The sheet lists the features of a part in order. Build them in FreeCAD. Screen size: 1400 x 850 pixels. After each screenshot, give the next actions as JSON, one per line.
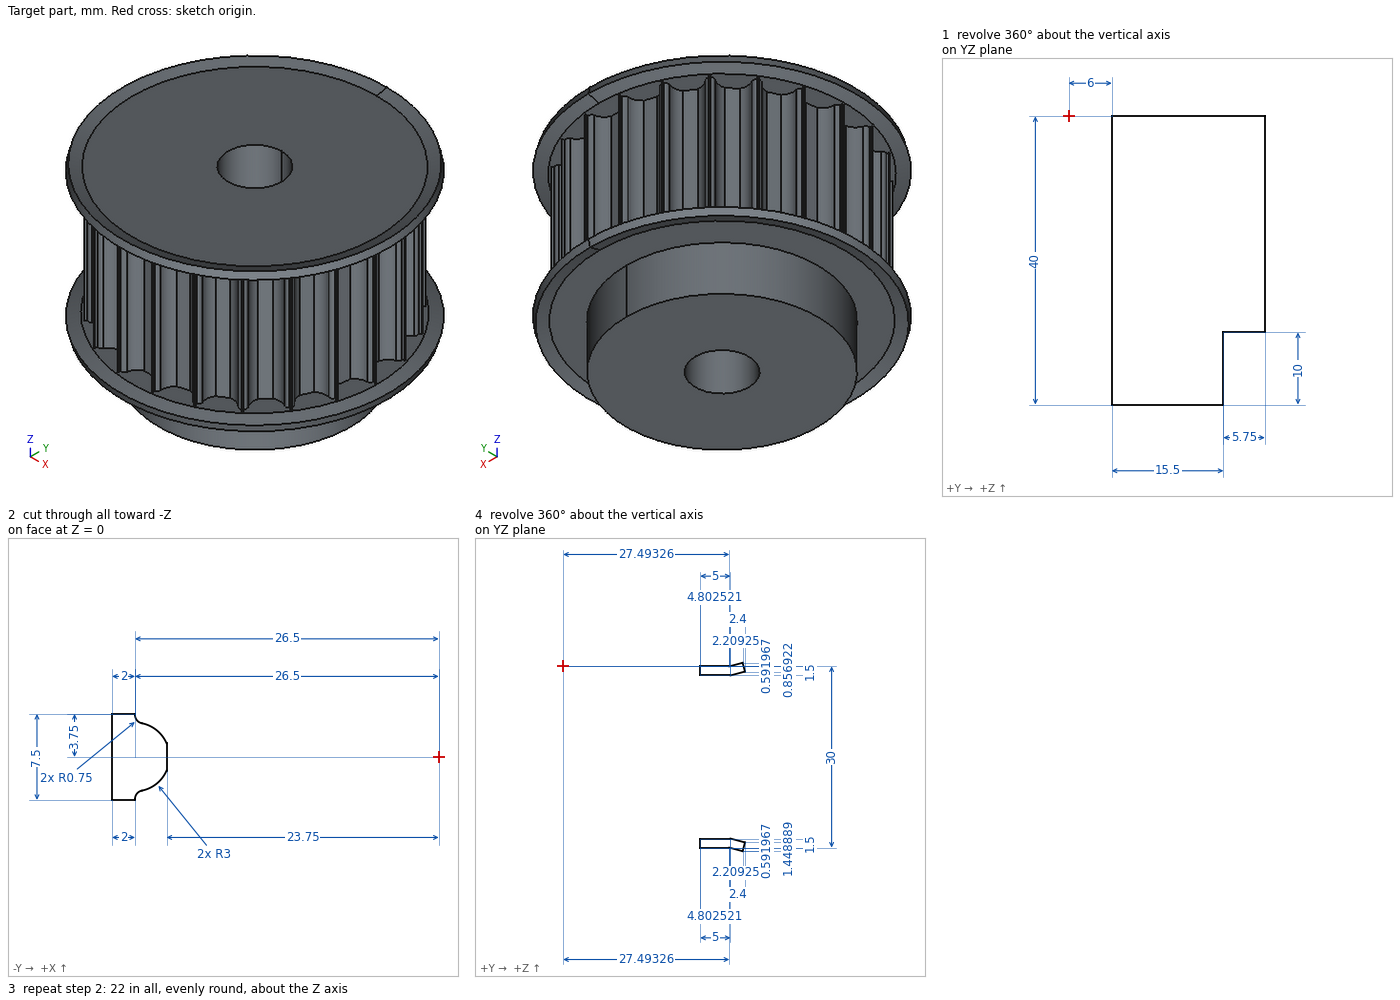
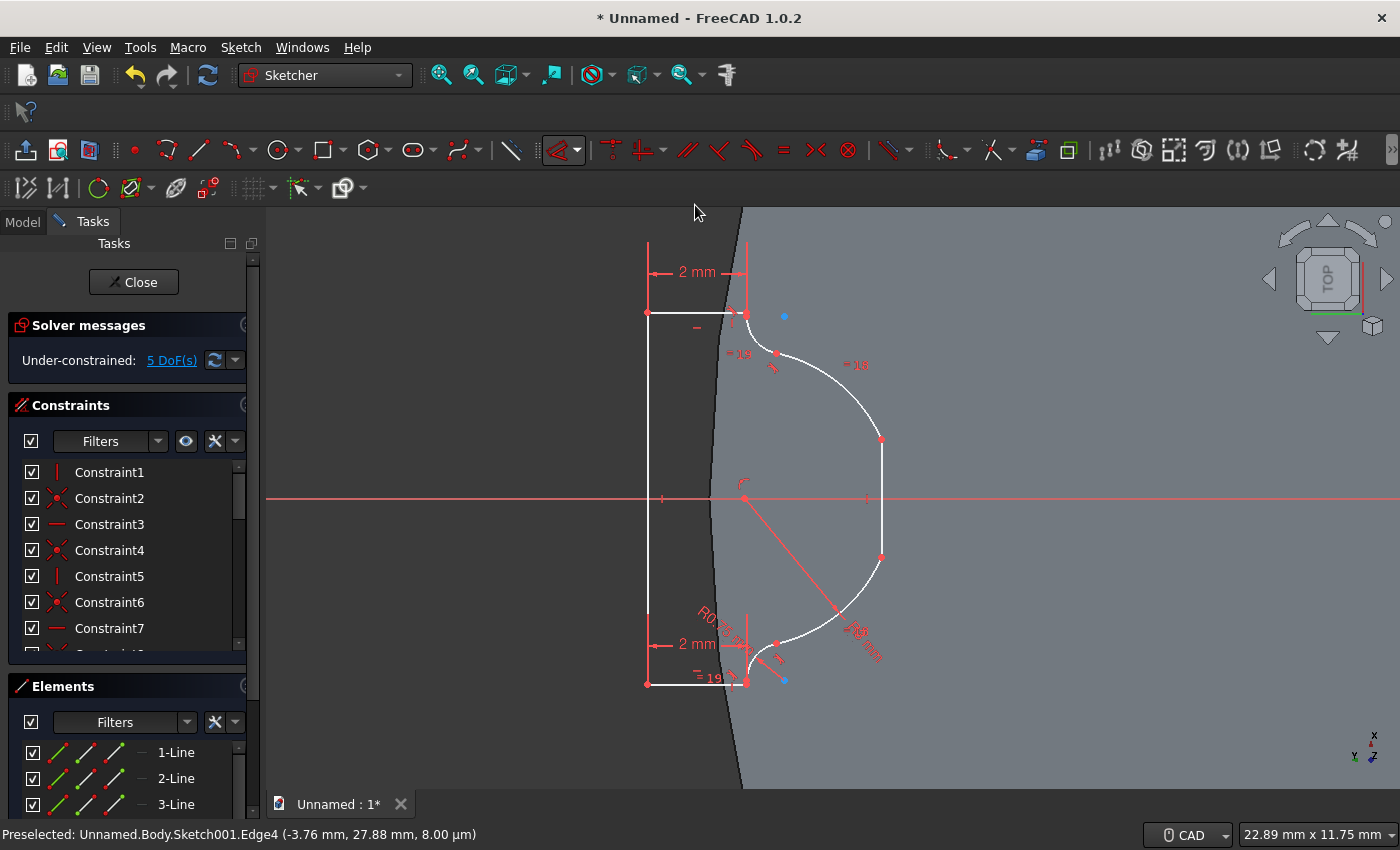
{"action": "left_click", "coordinate": [648, 425]}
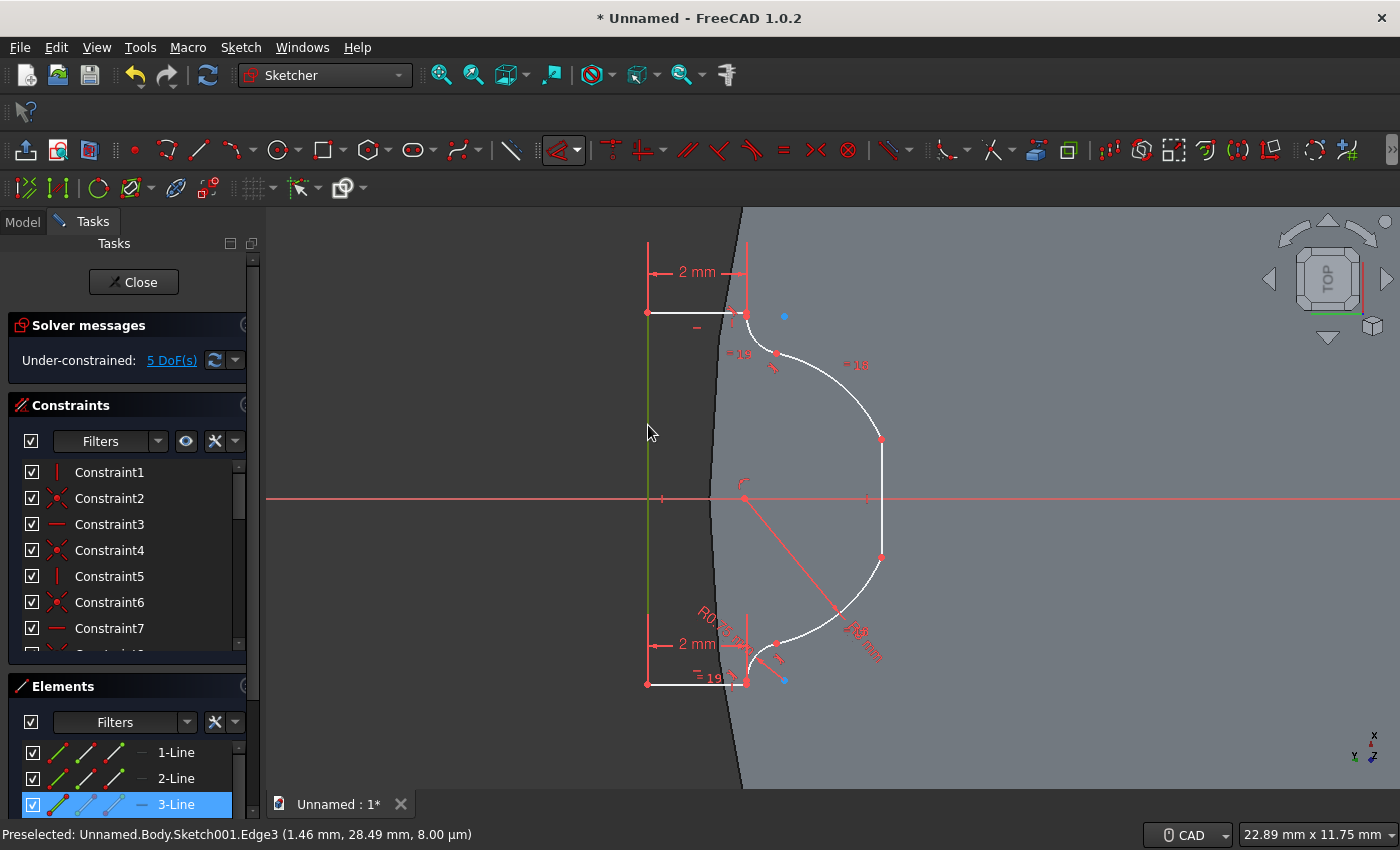
{"action": "key", "text": "i"}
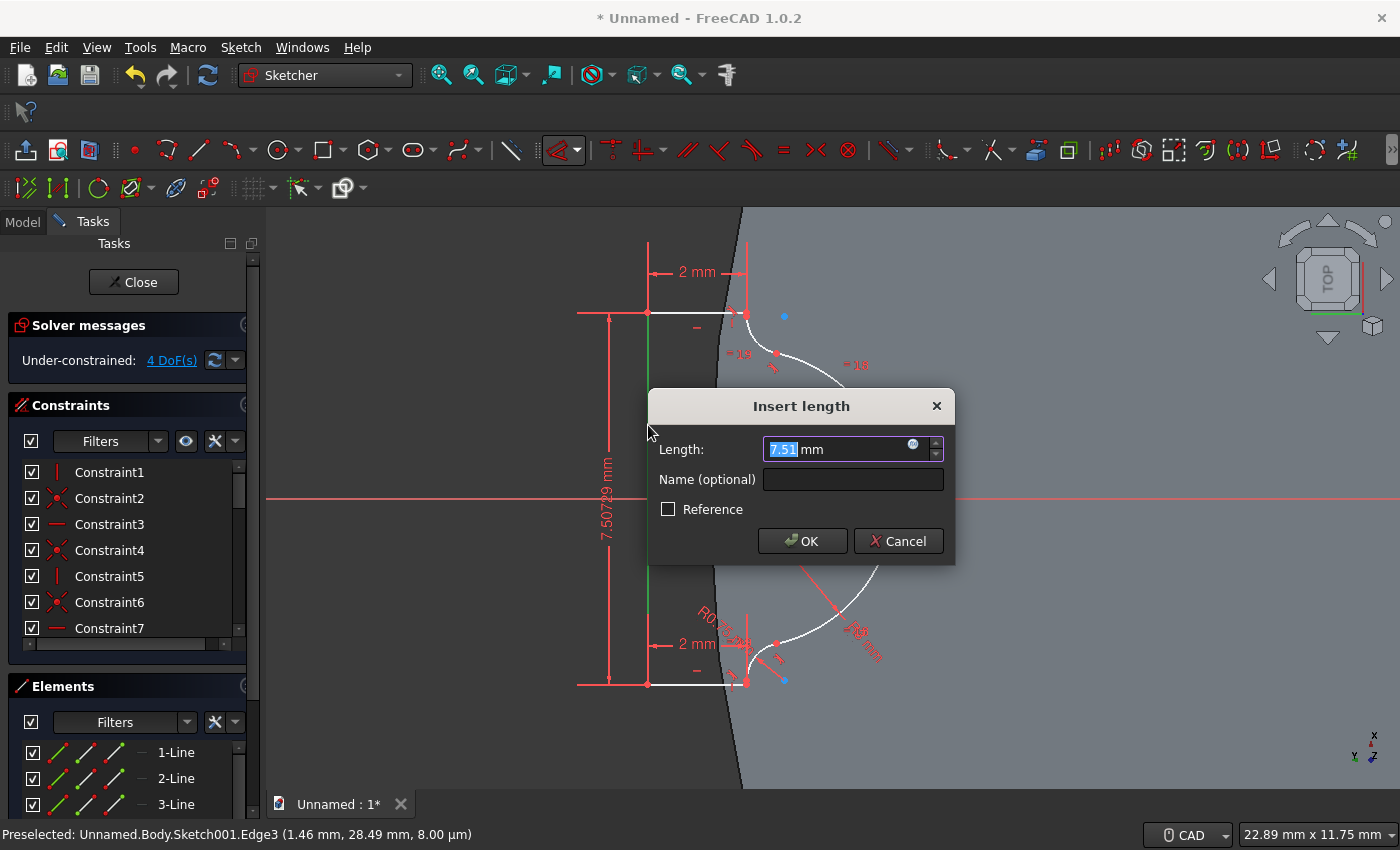
{"action": "type", "text": "7.5"}
{"action": "key", "text": "Return"}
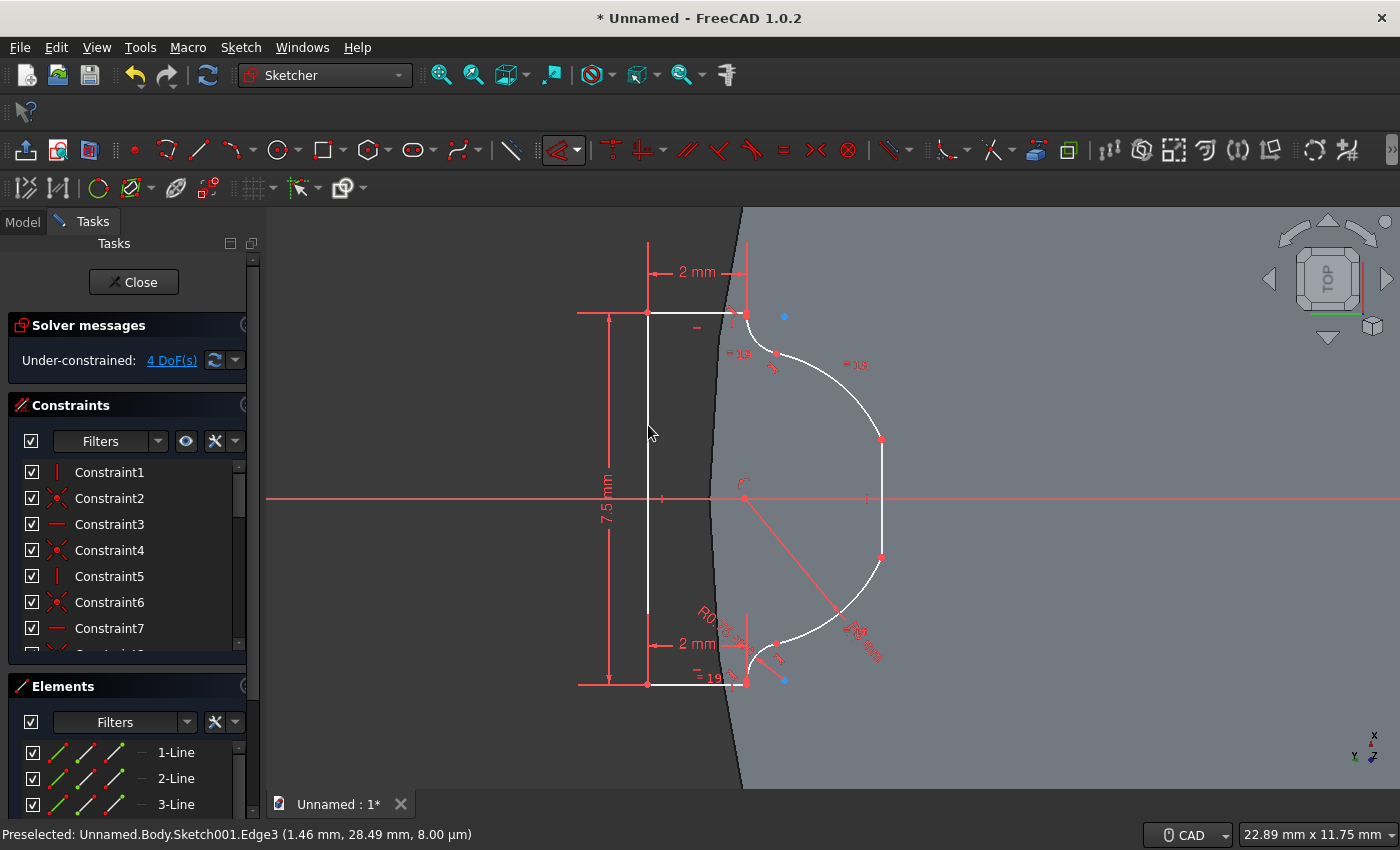
{"action": "scroll", "coordinate": [747, 317], "scroll_direction": "up", "scroll_amount": 6}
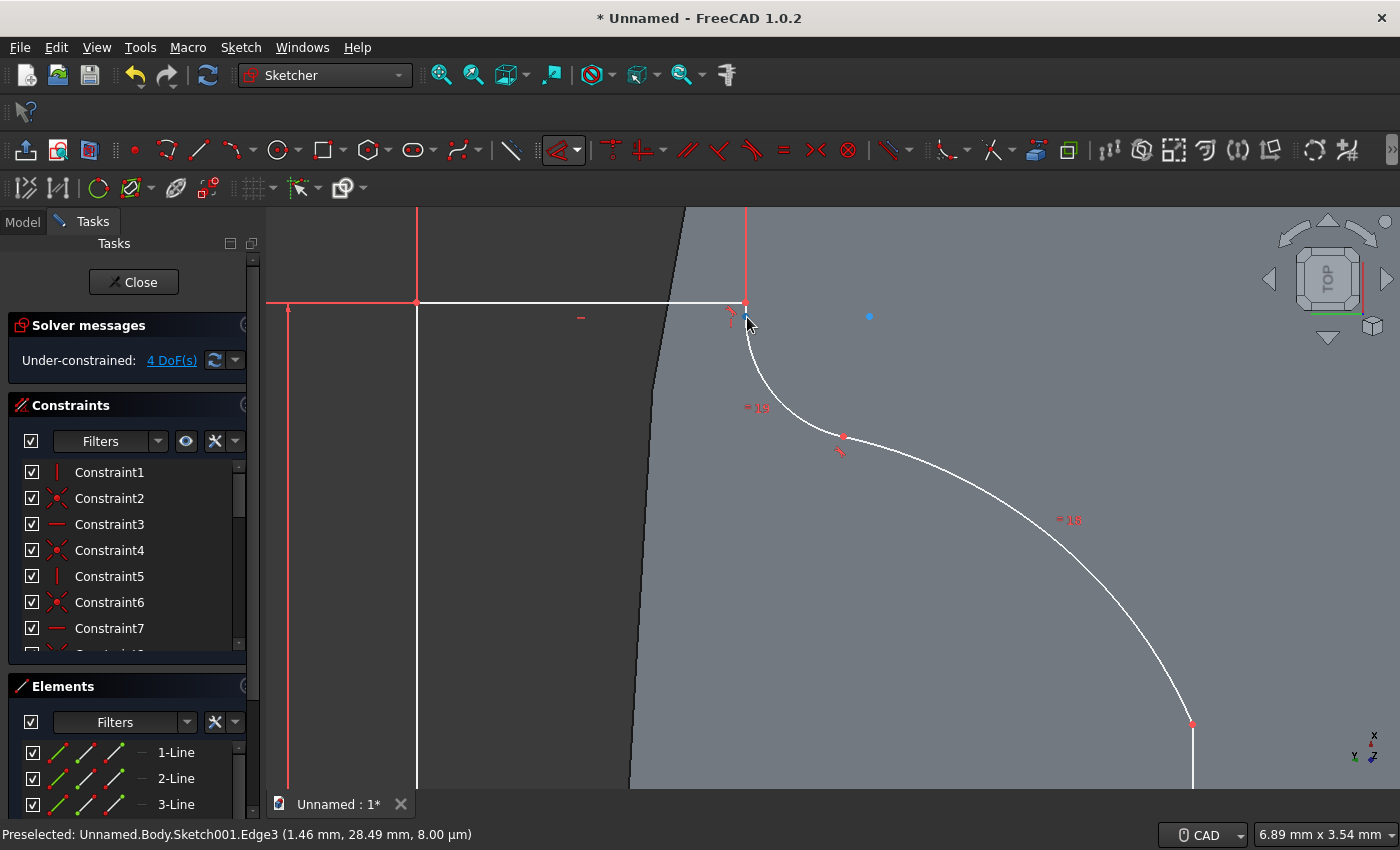
{"action": "left_click", "coordinate": [746, 316]}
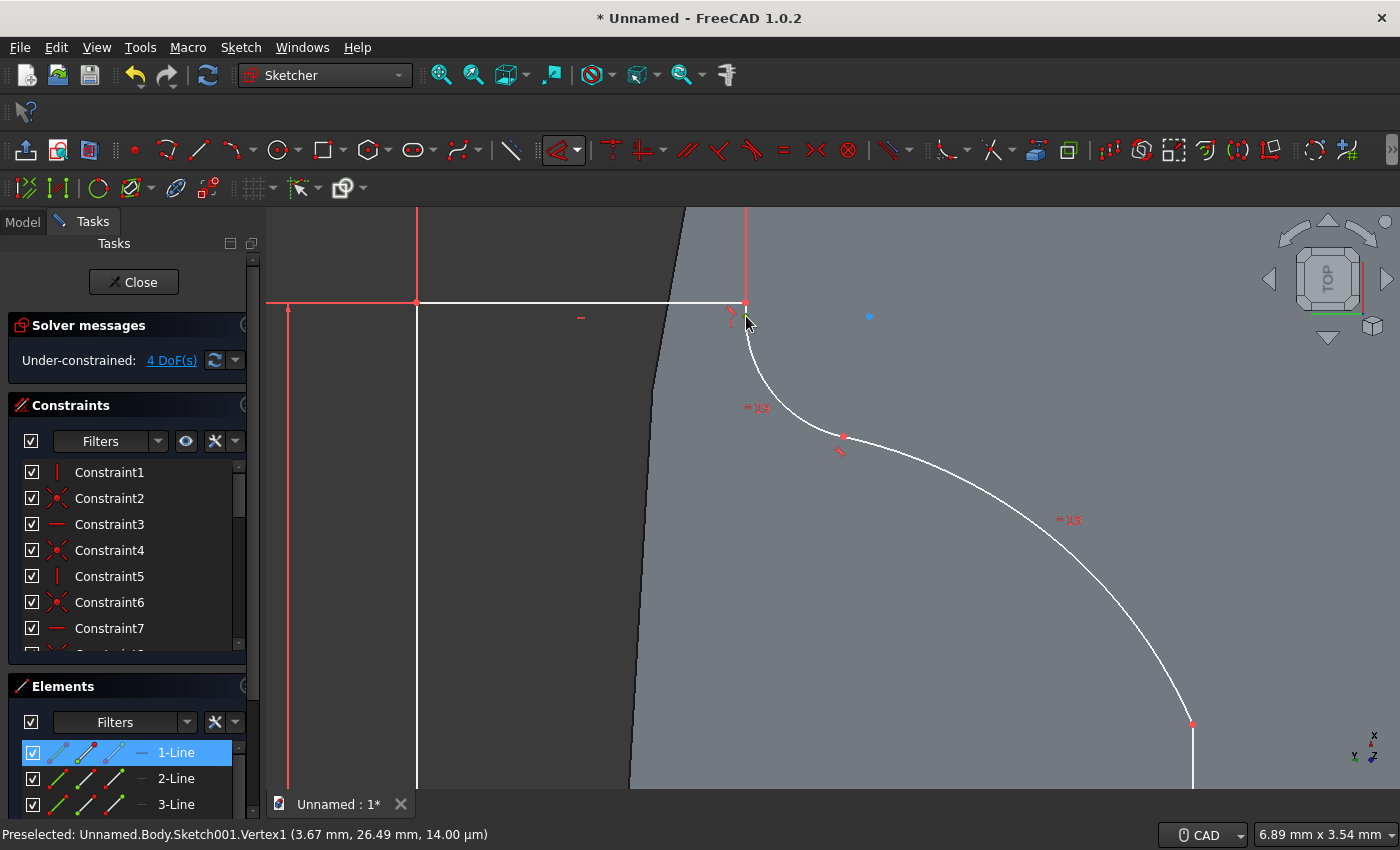
{"action": "key", "text": "l"}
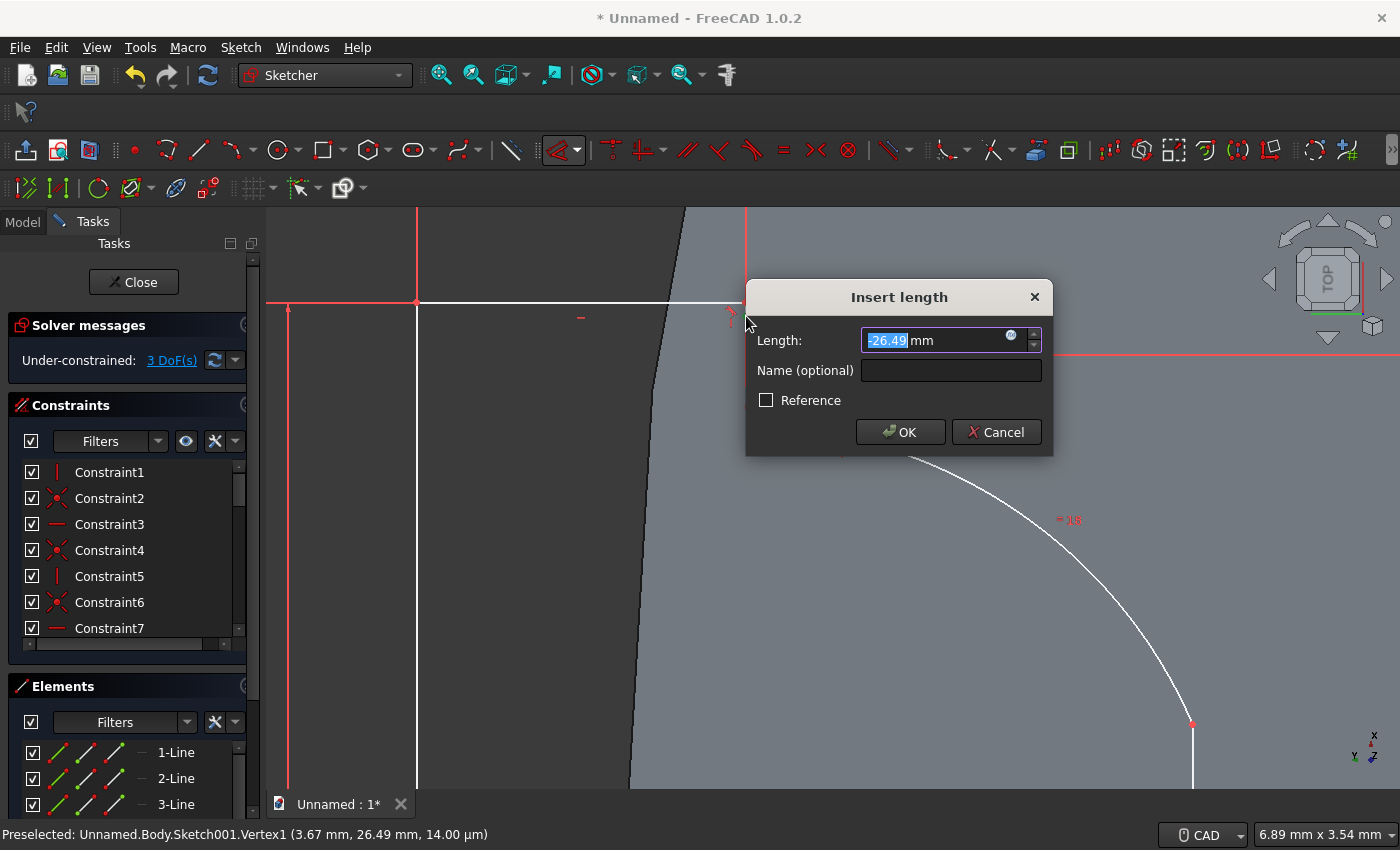
{"action": "type", "text": "-26.5"}
{"action": "key", "text": "Return"}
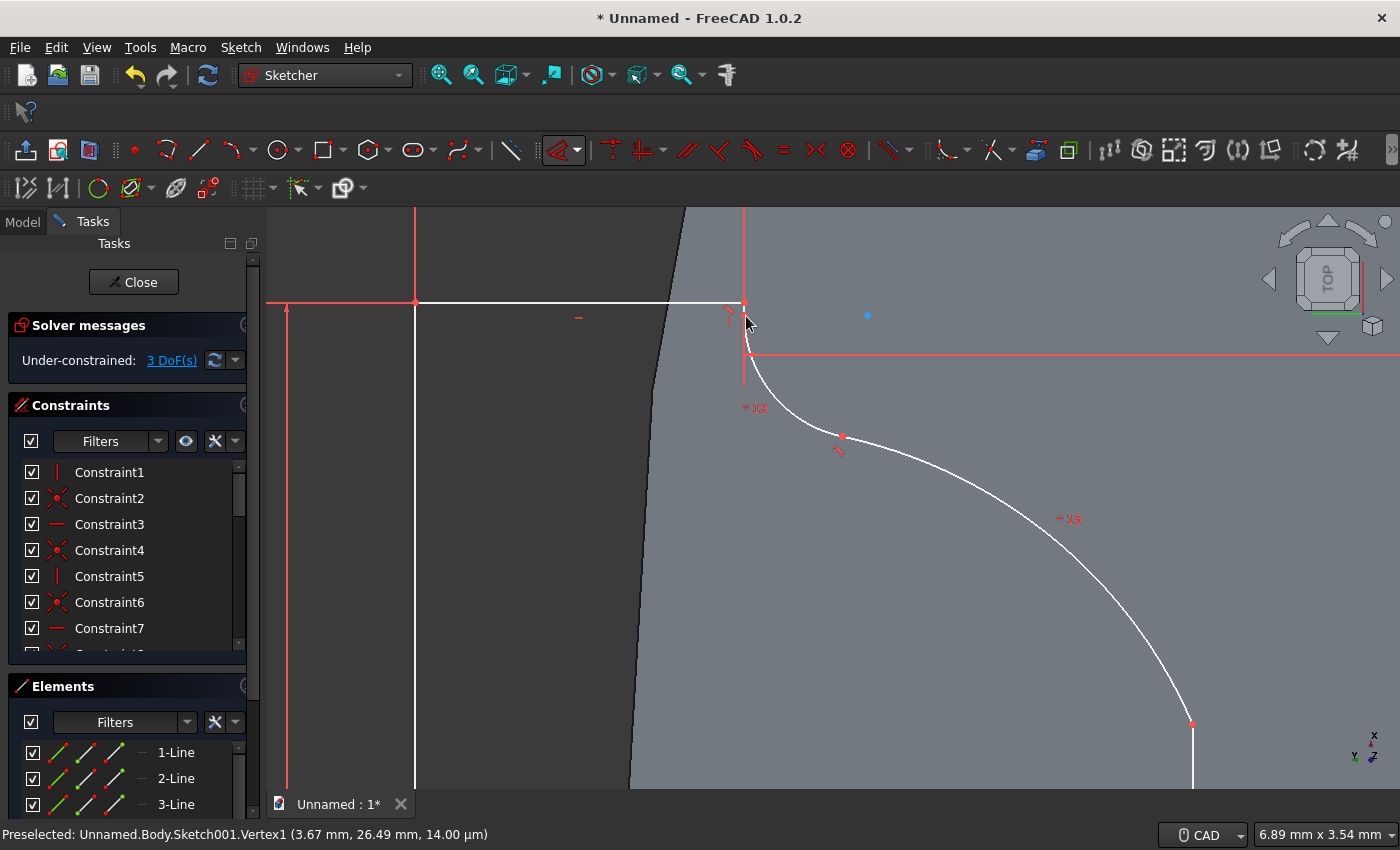
{"action": "left_click", "coordinate": [744, 303]}